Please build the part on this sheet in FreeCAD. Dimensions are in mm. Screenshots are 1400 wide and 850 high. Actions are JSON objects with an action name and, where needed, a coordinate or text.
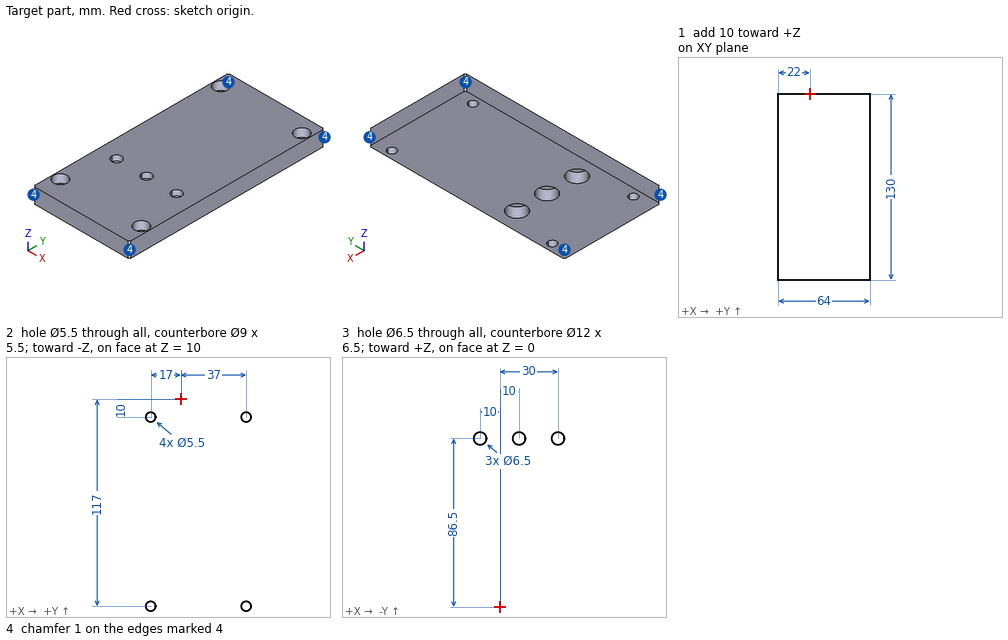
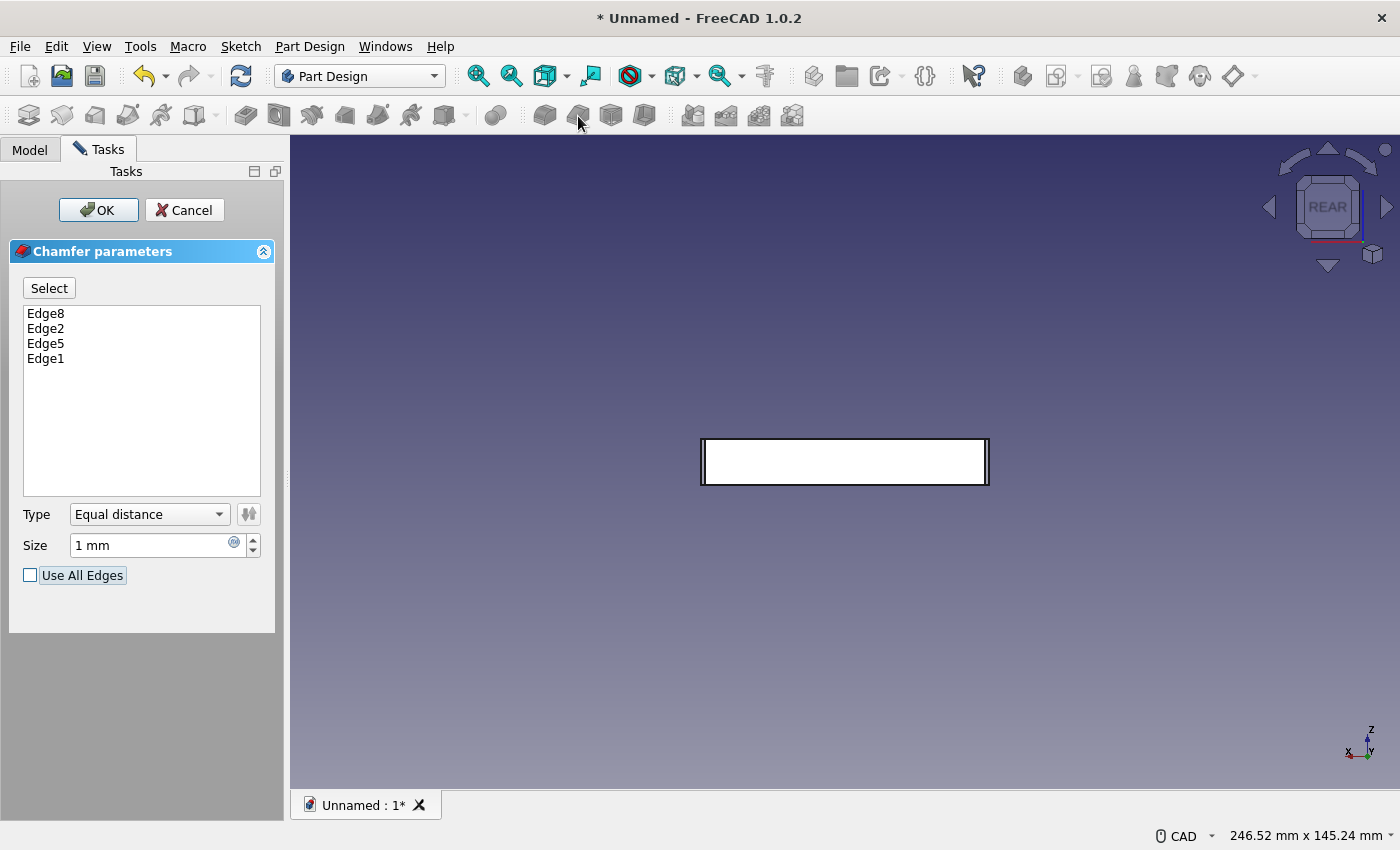
{"action": "left_click", "coordinate": [99, 210]}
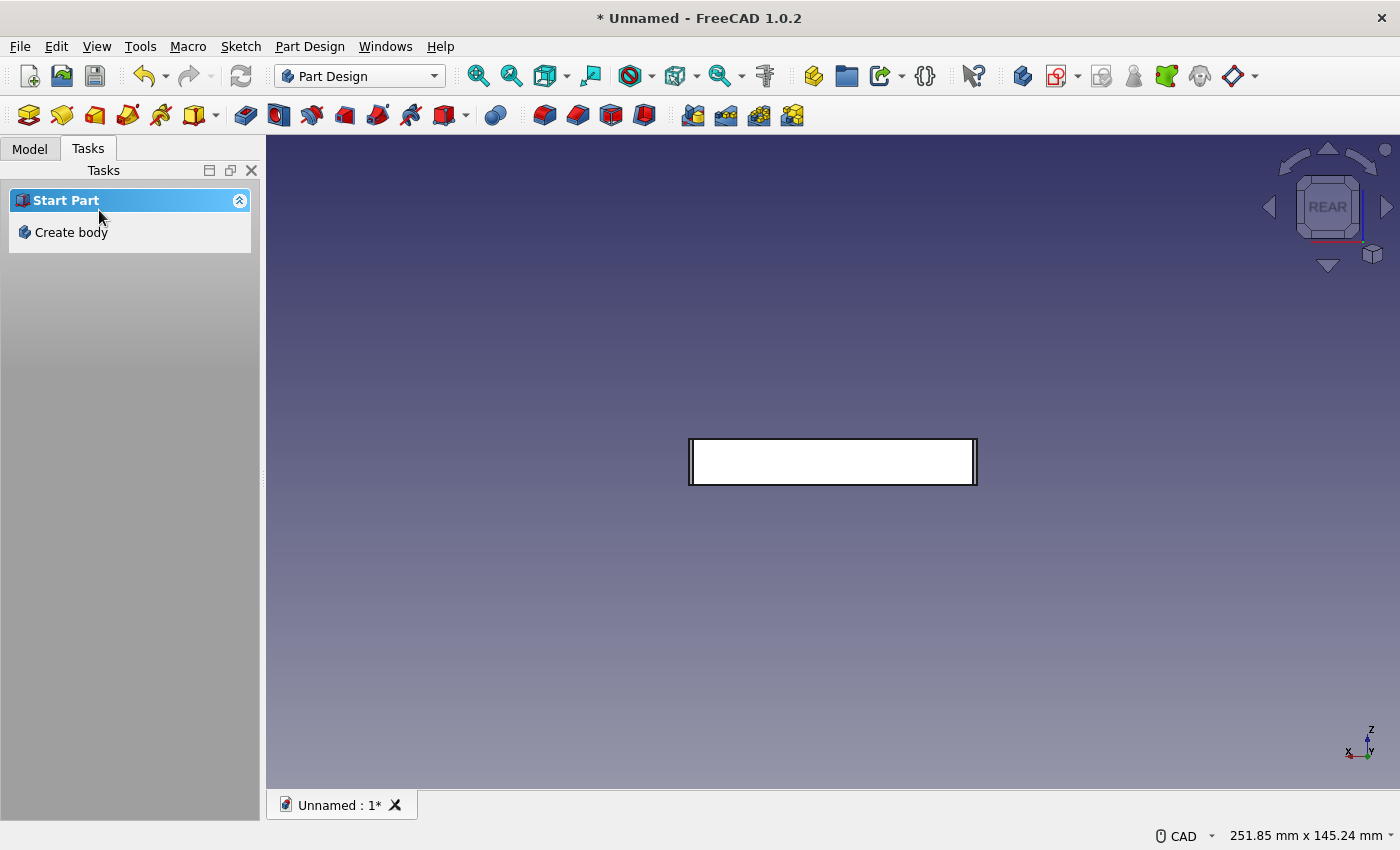
{"action": "key", "text": "0"}